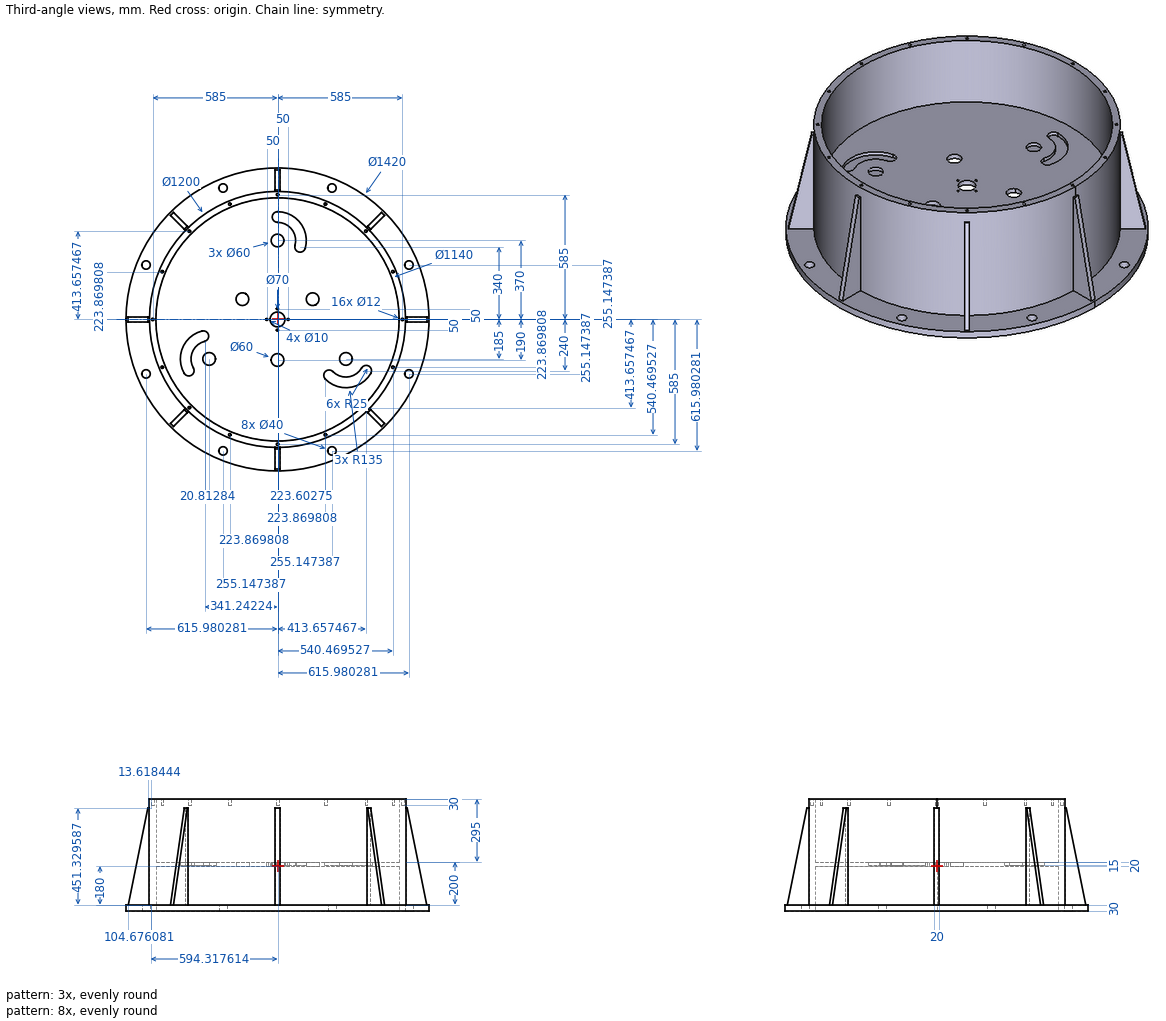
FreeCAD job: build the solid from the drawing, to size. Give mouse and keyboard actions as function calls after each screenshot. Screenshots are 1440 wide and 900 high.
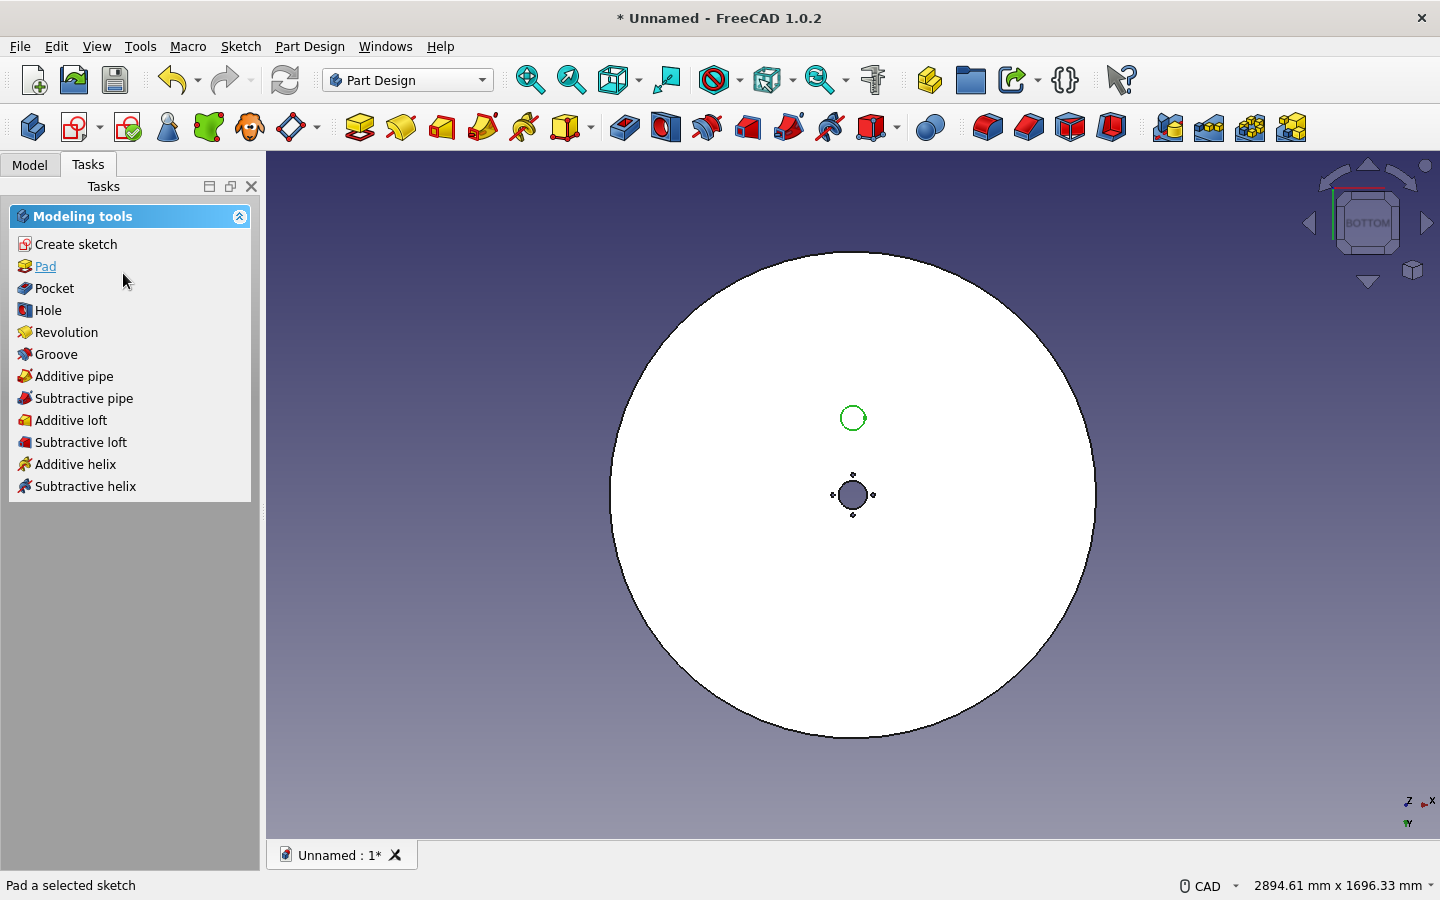
click(625, 128)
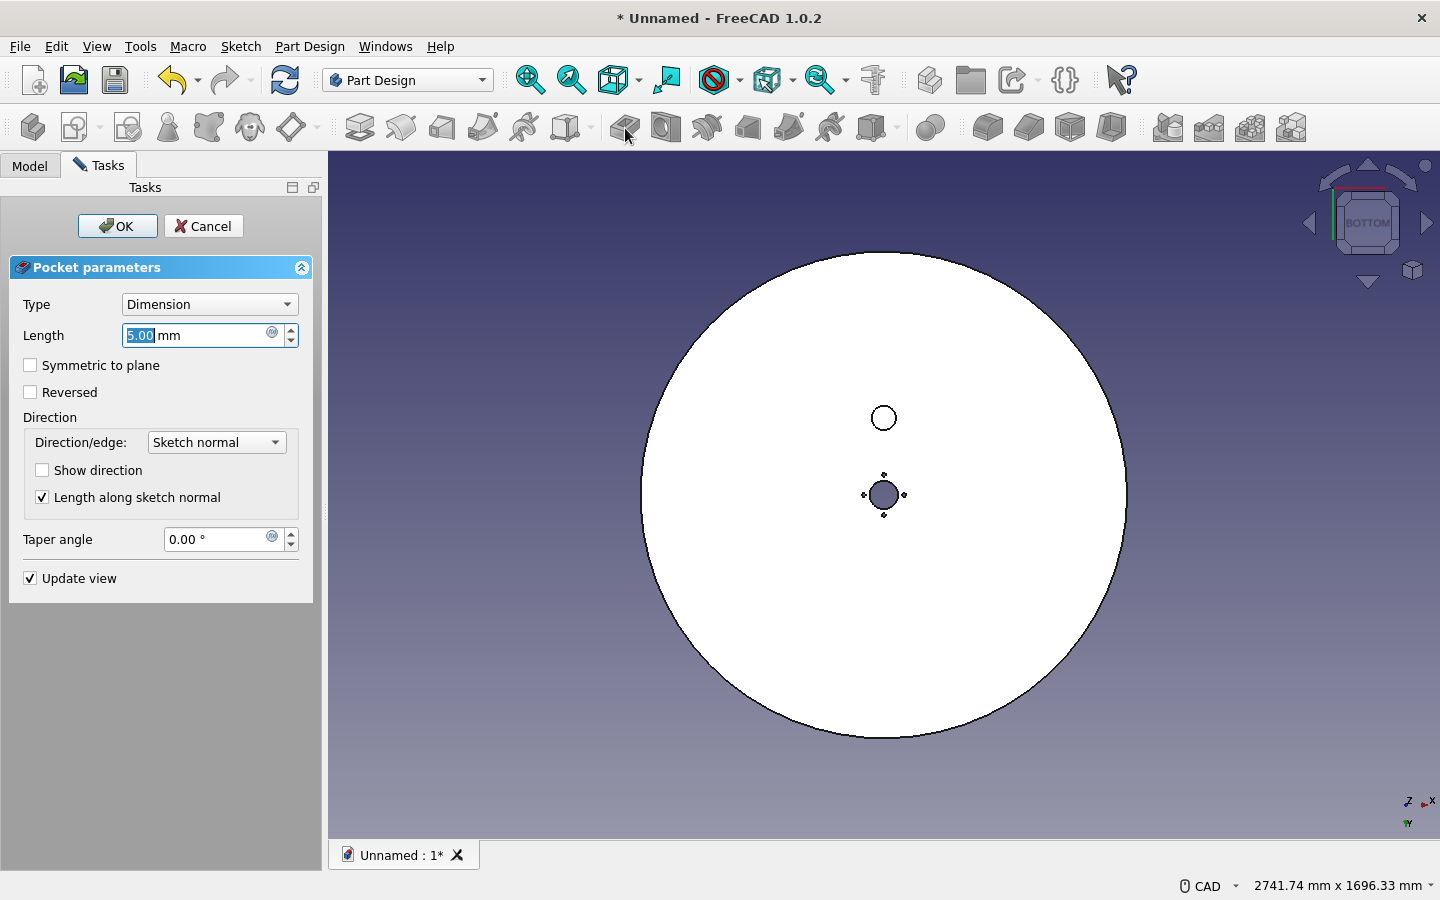
click(210, 304)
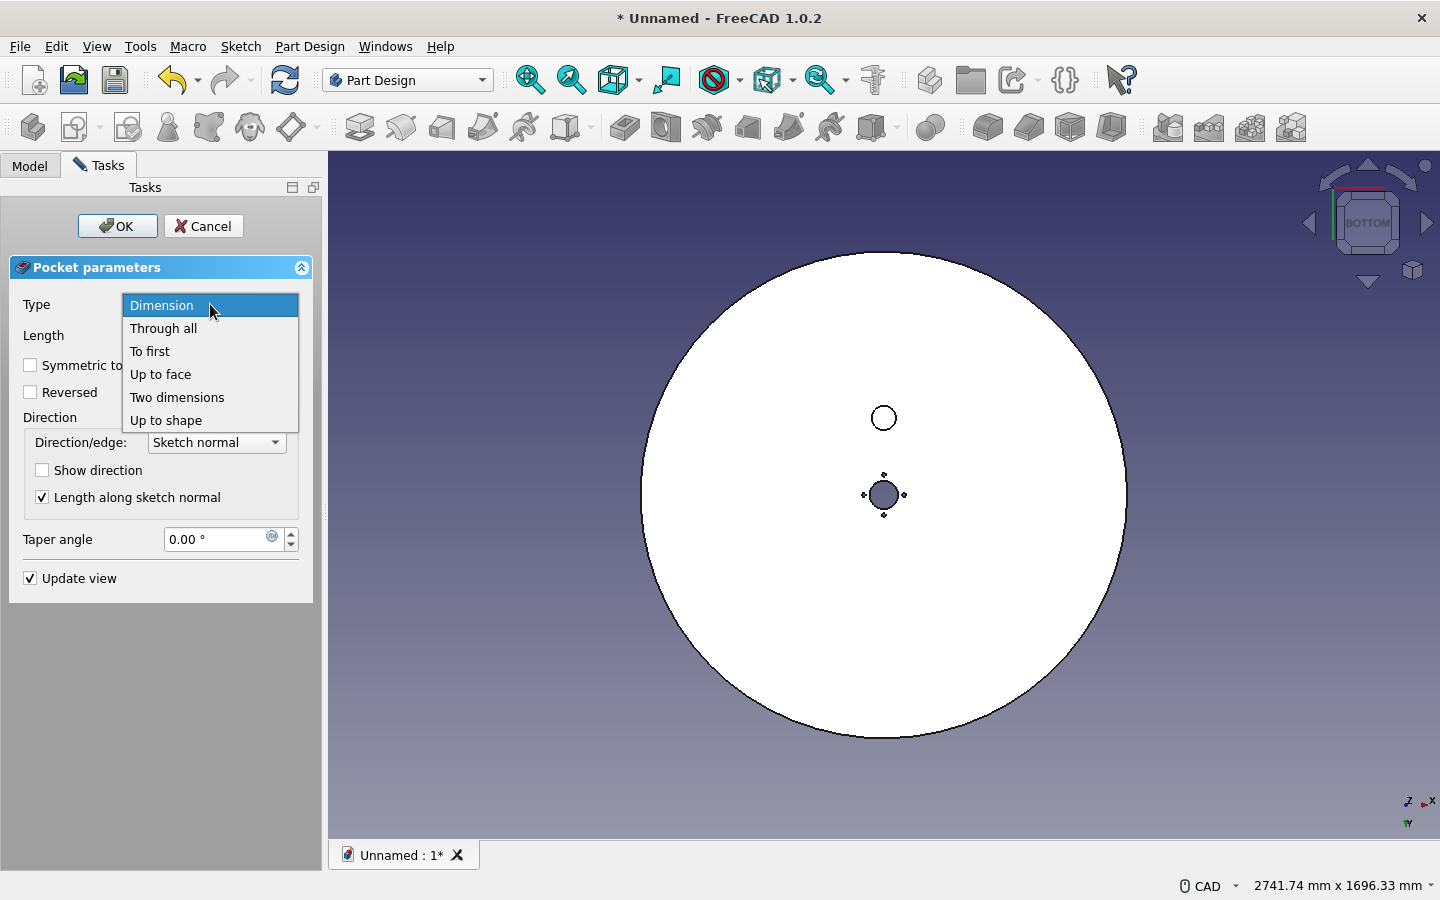
click(208, 328)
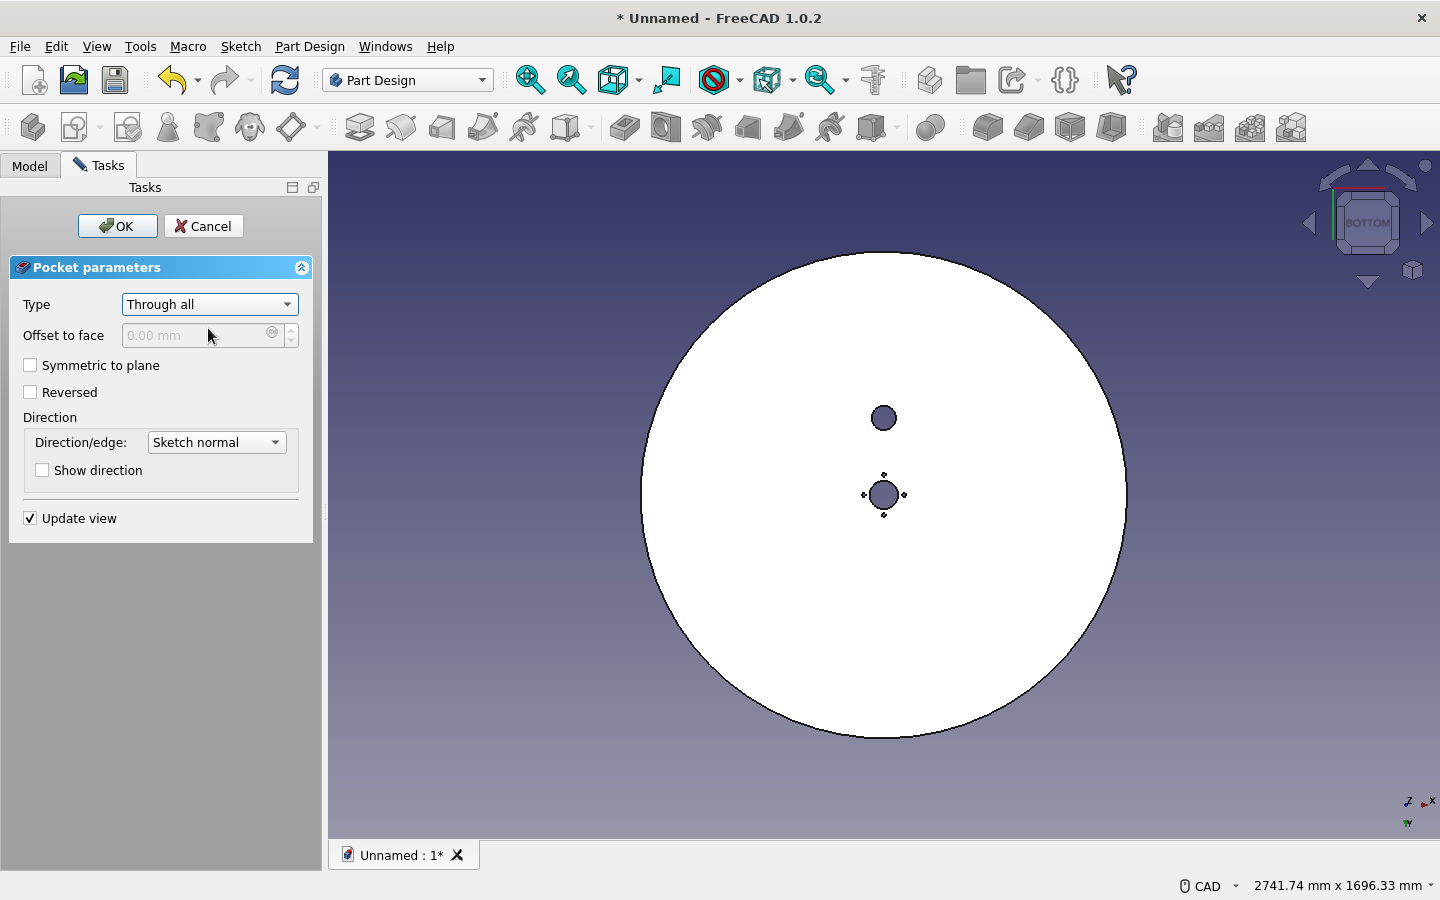
click(118, 226)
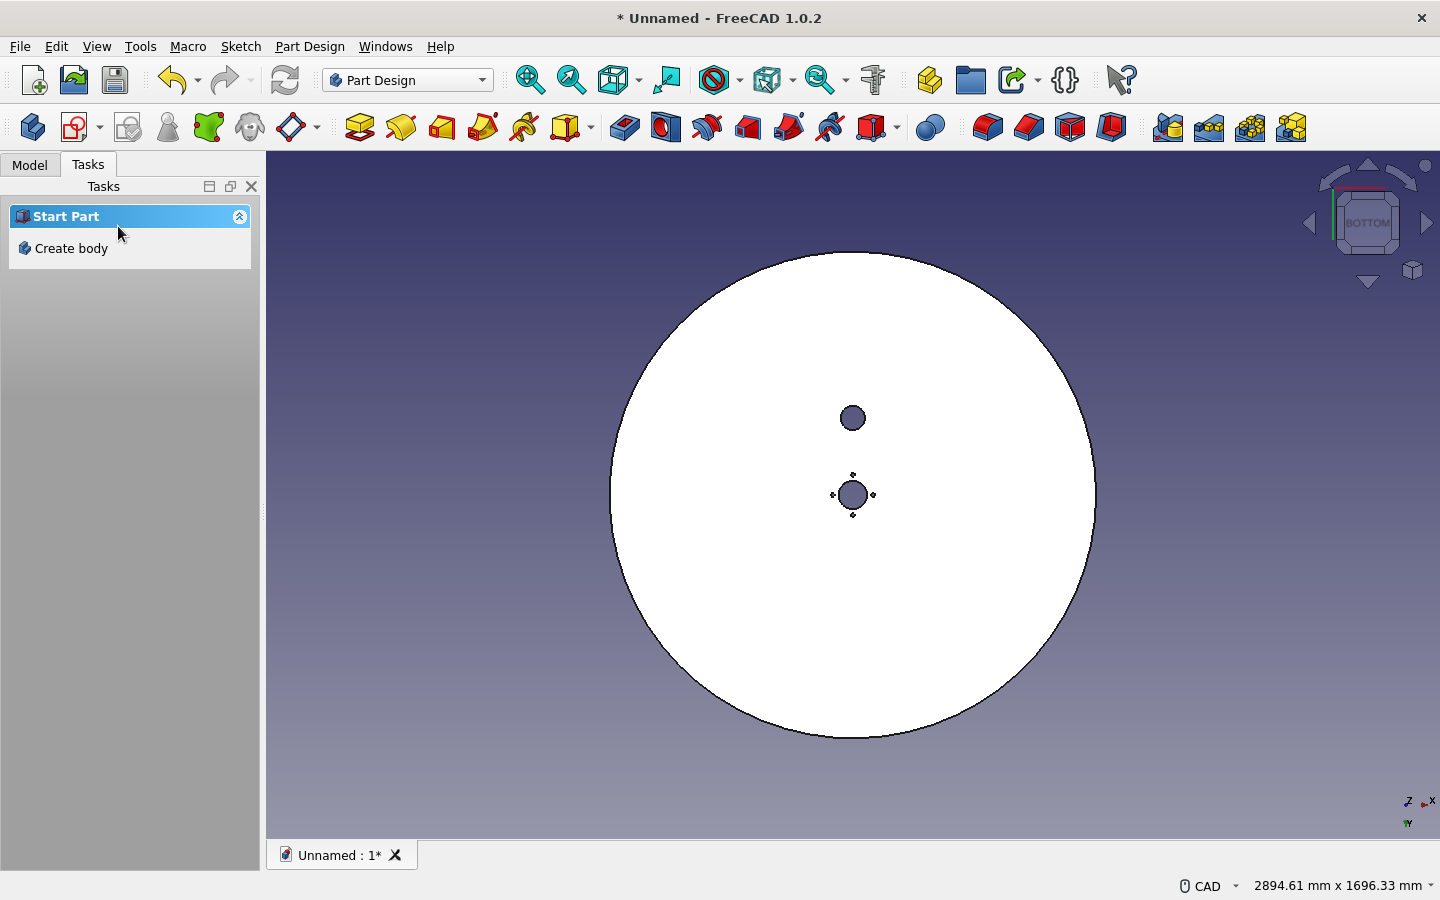
click(30, 164)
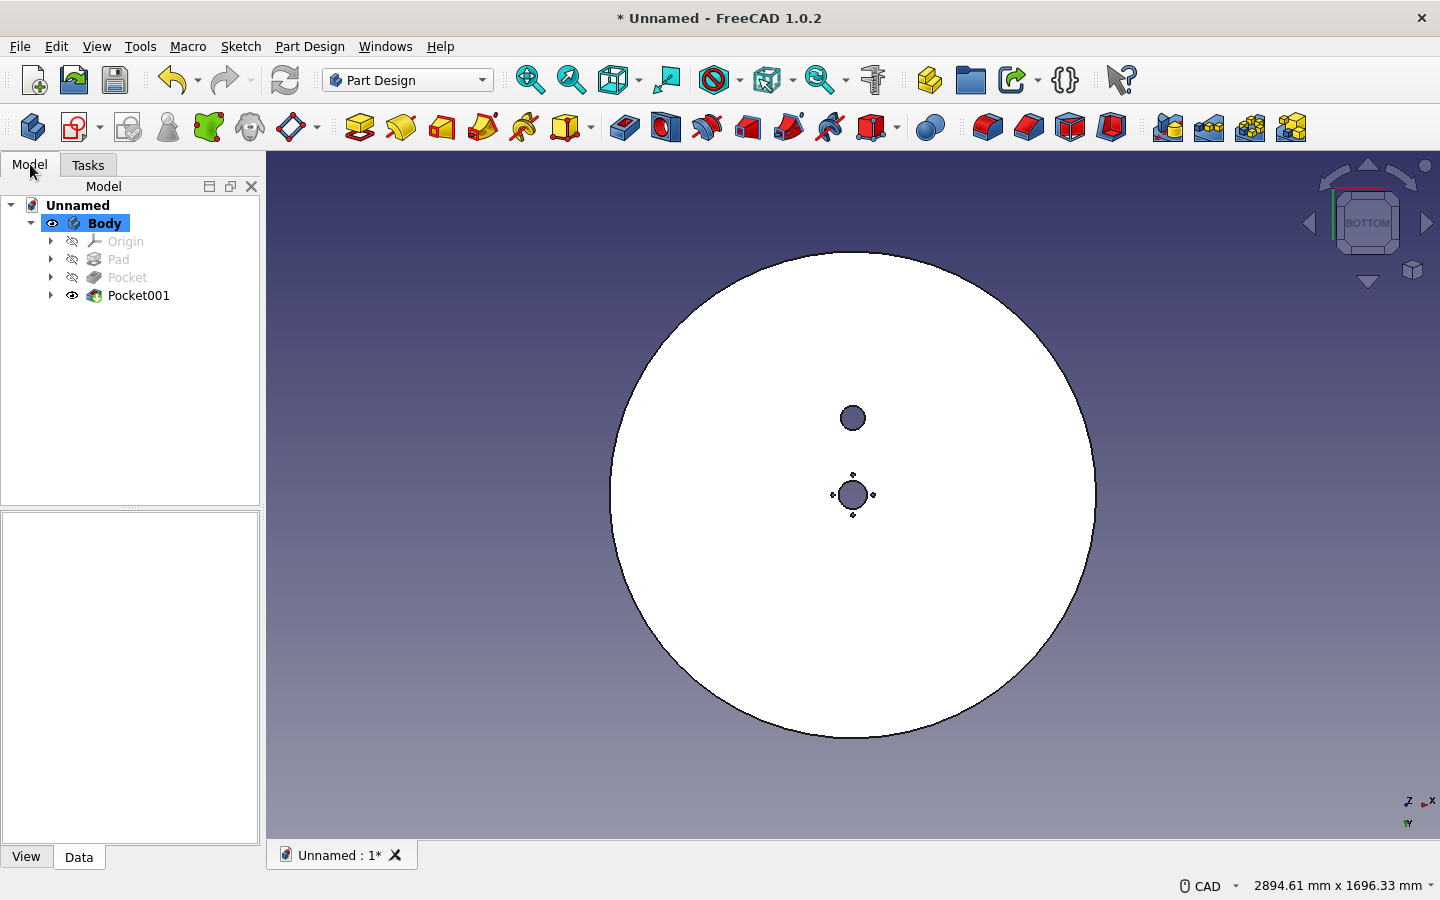
click(117, 295)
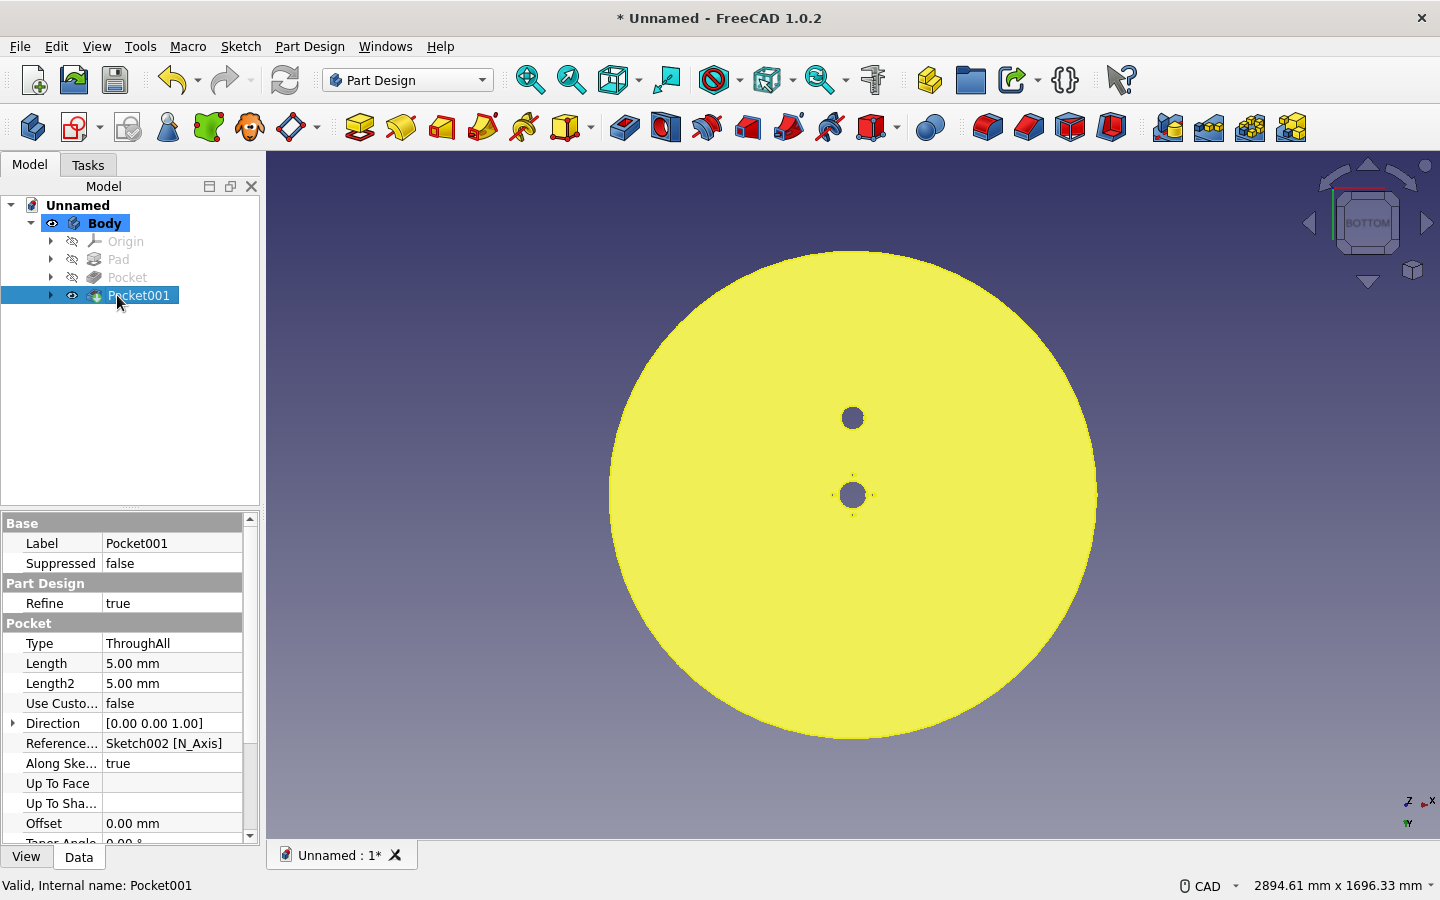
click(1250, 128)